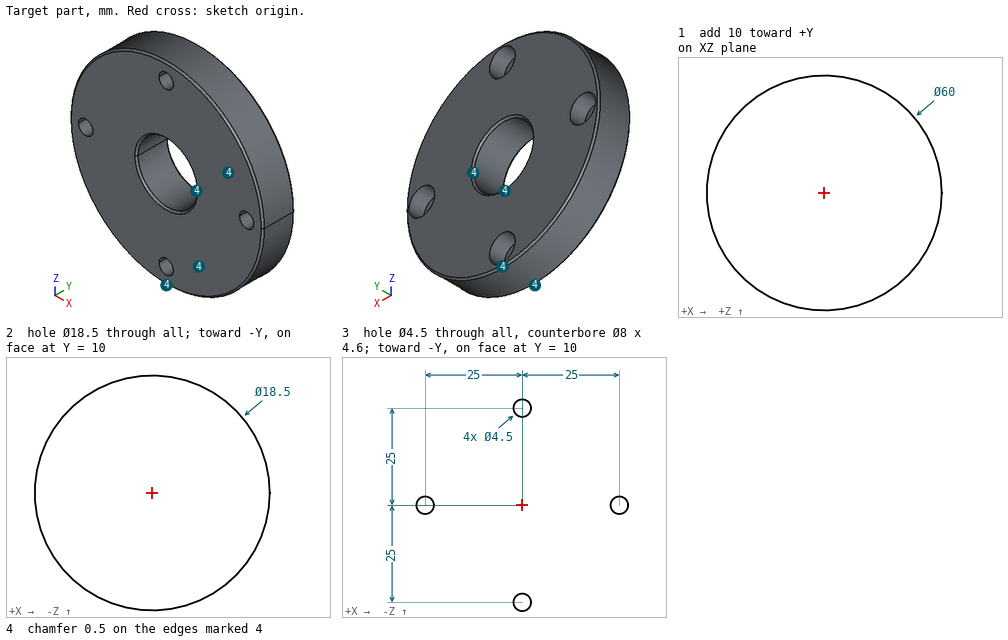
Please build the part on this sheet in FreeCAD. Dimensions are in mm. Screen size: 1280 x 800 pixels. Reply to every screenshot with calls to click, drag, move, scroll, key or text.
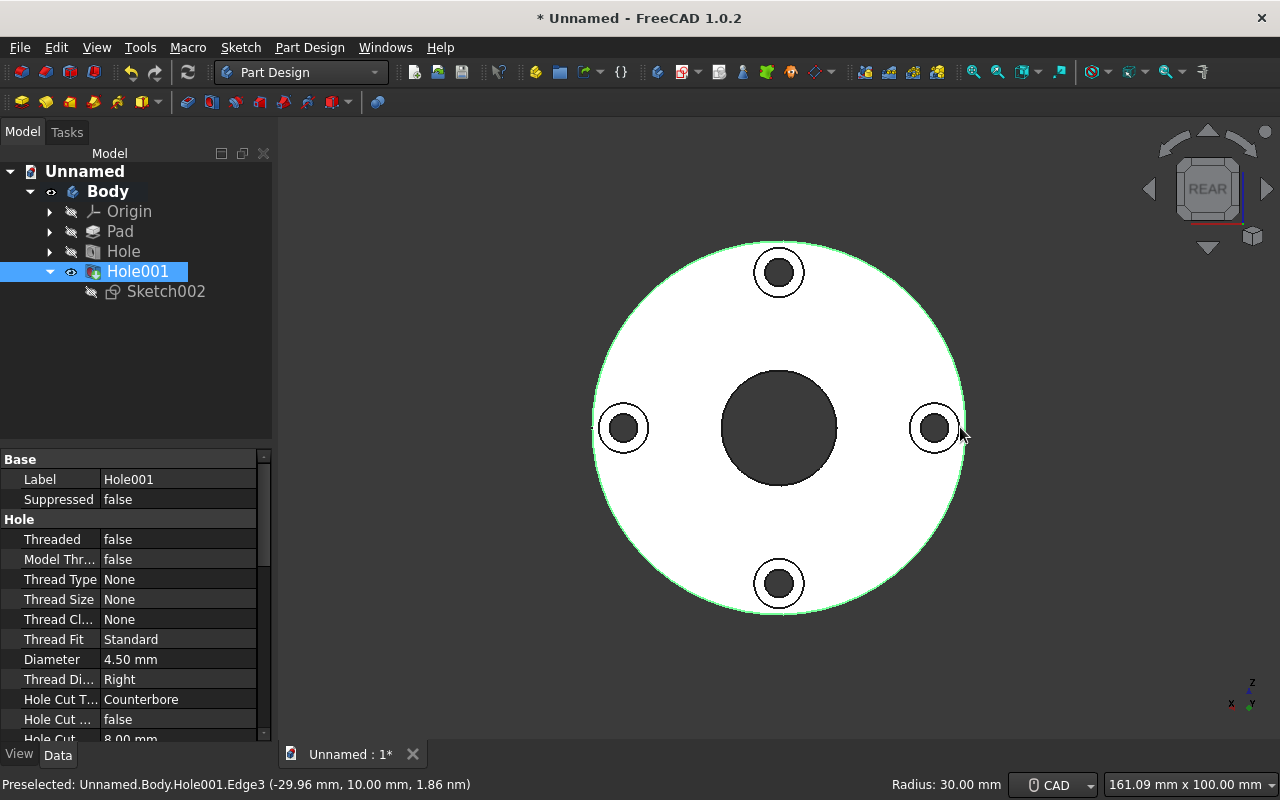
click(721, 427, ctrl)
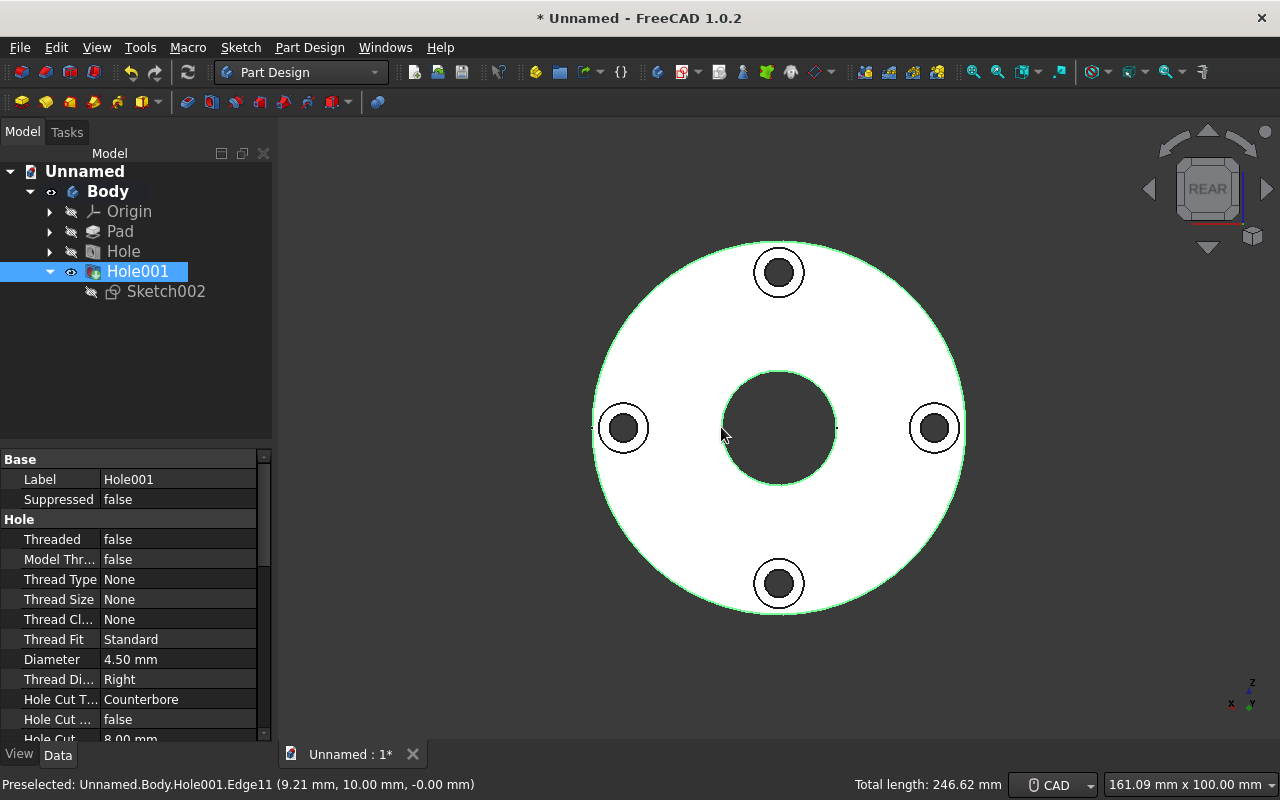
key(0)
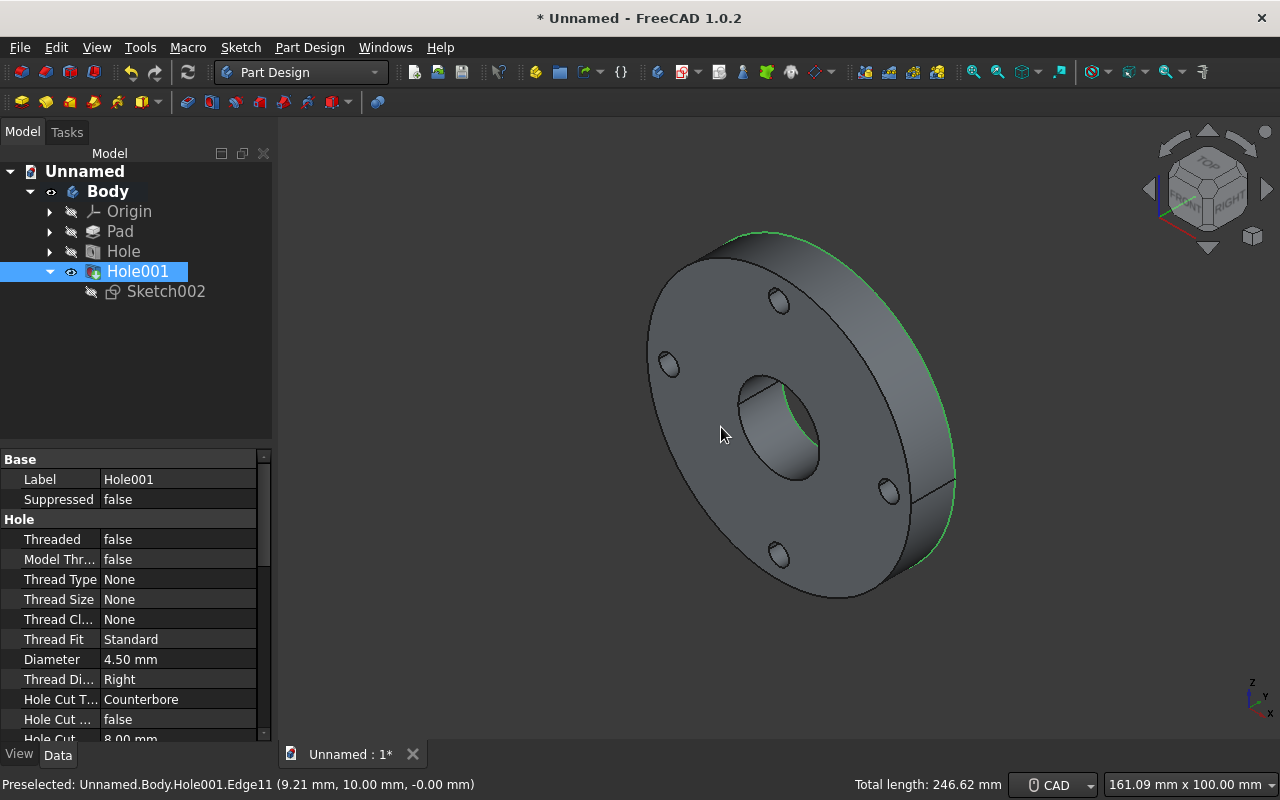
click(738, 259, ctrl)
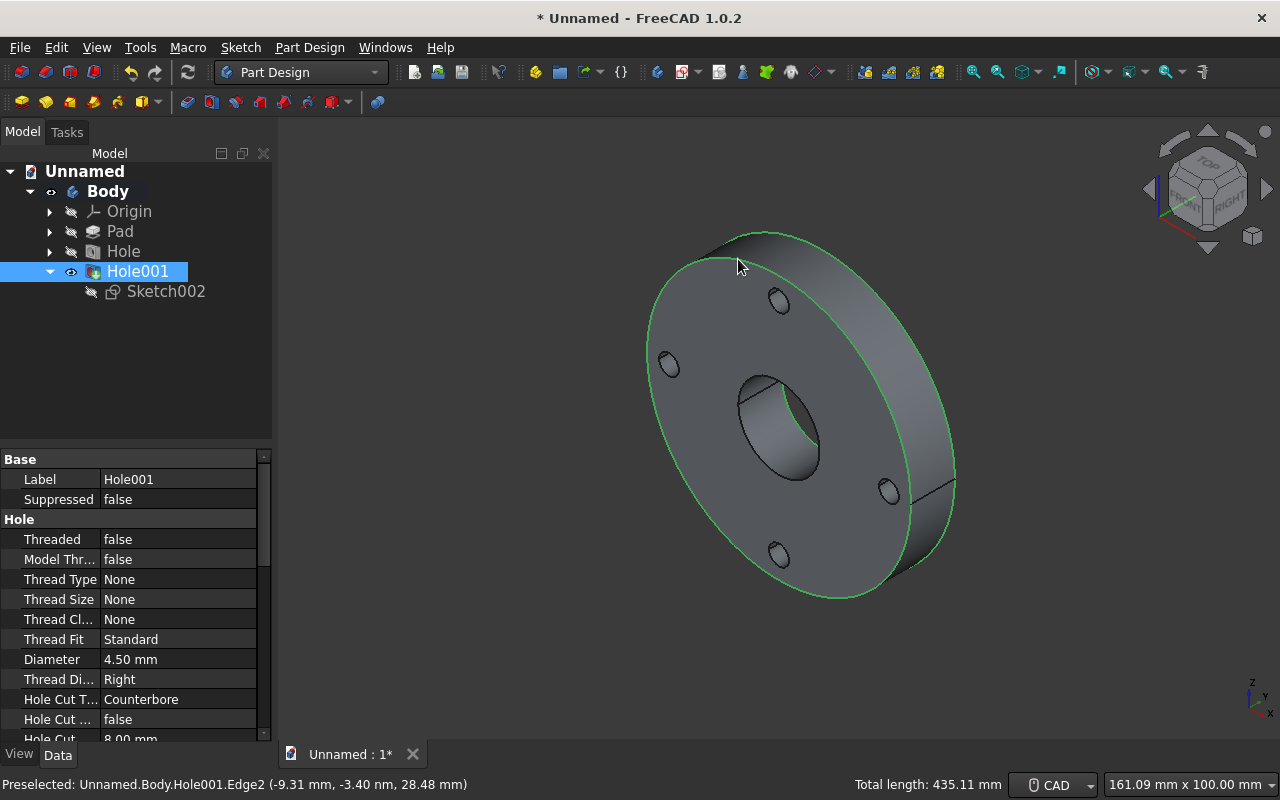
click(792, 479, ctrl)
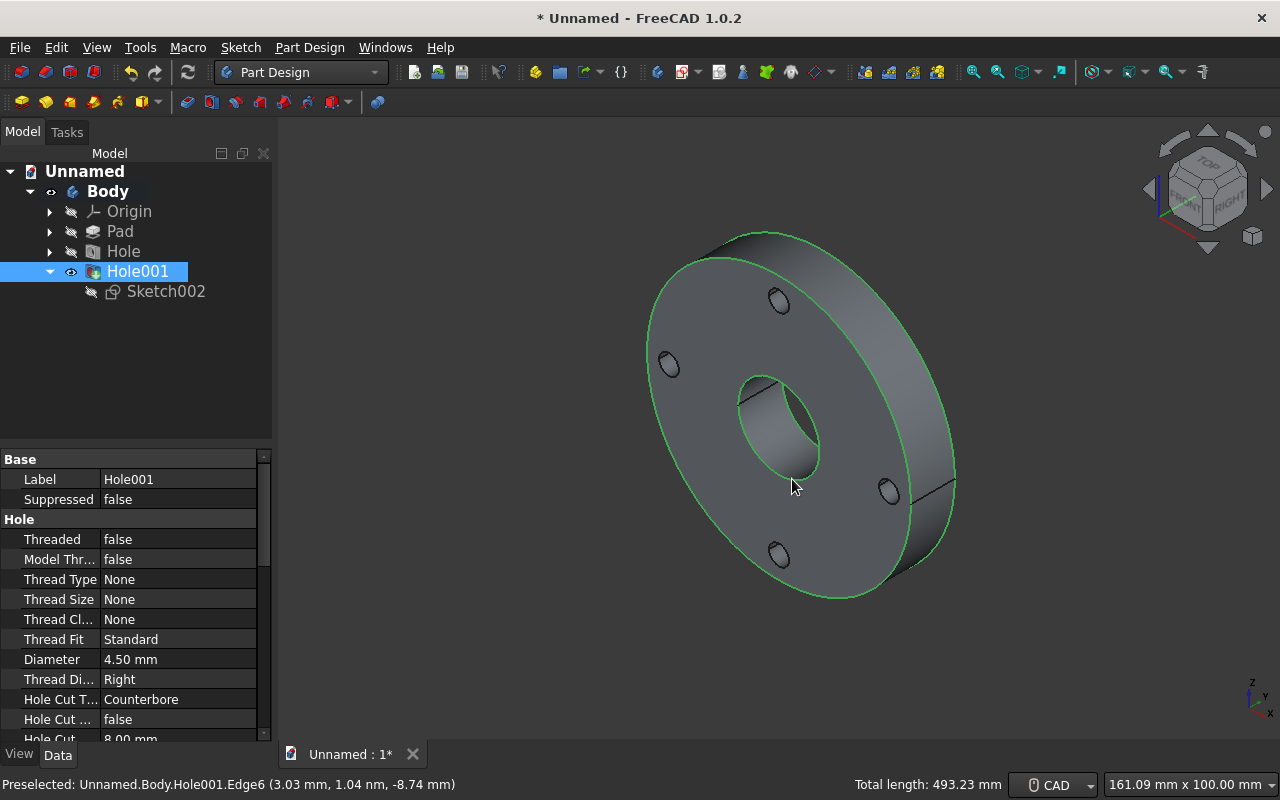
click(46, 72)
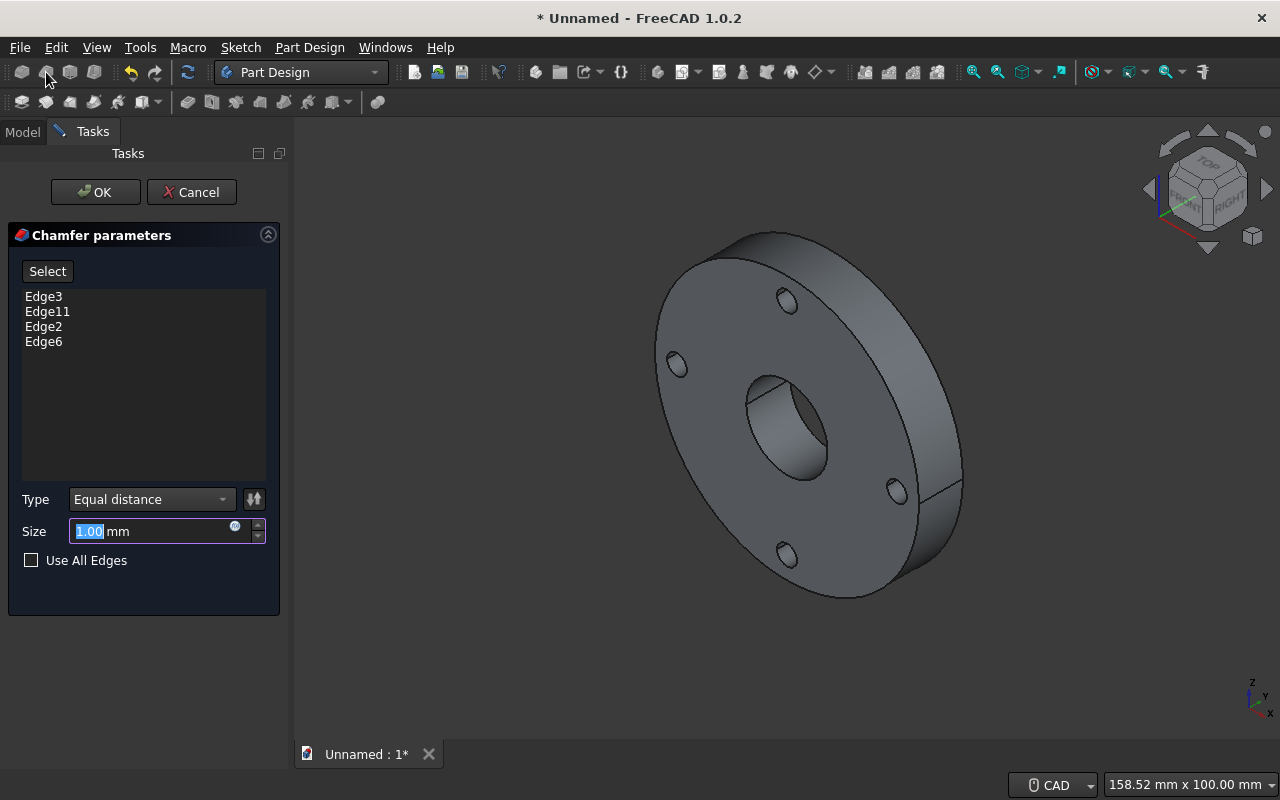
text(0.5)
key(Tab)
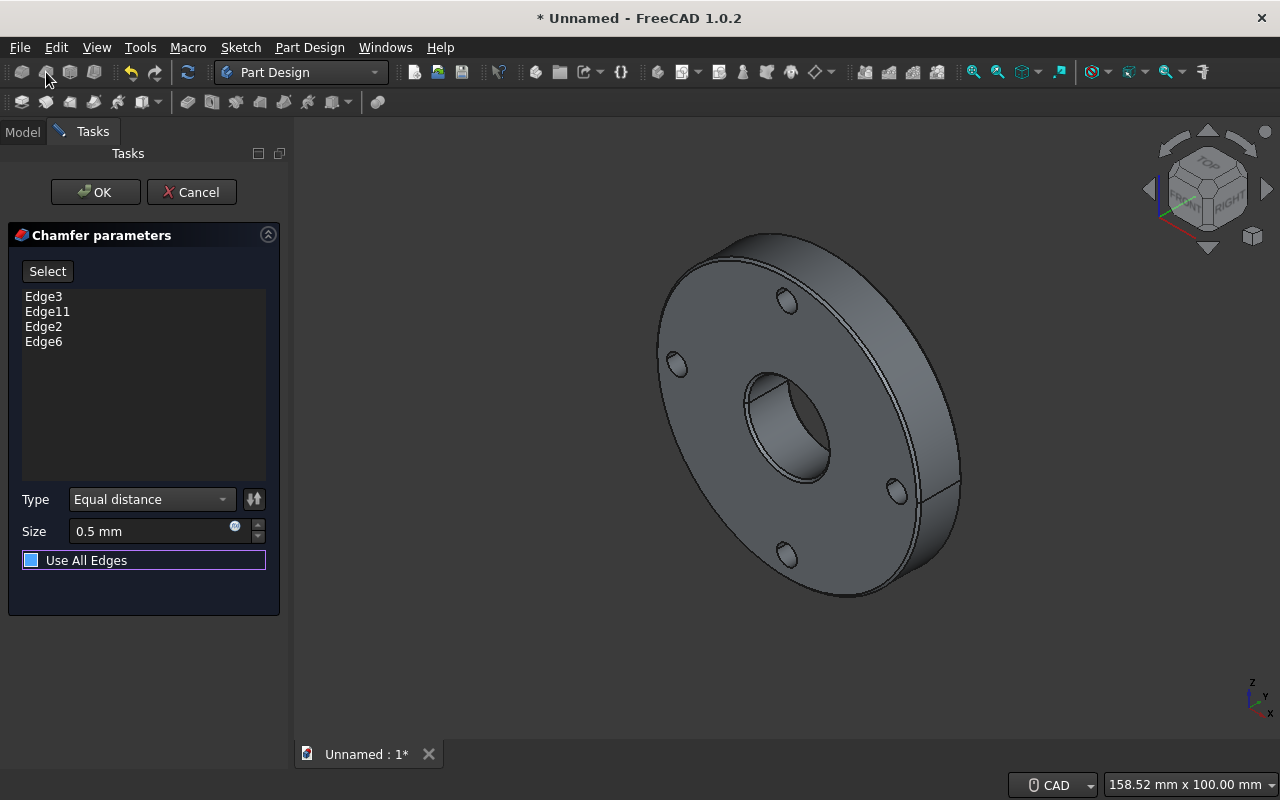
click(96, 192)